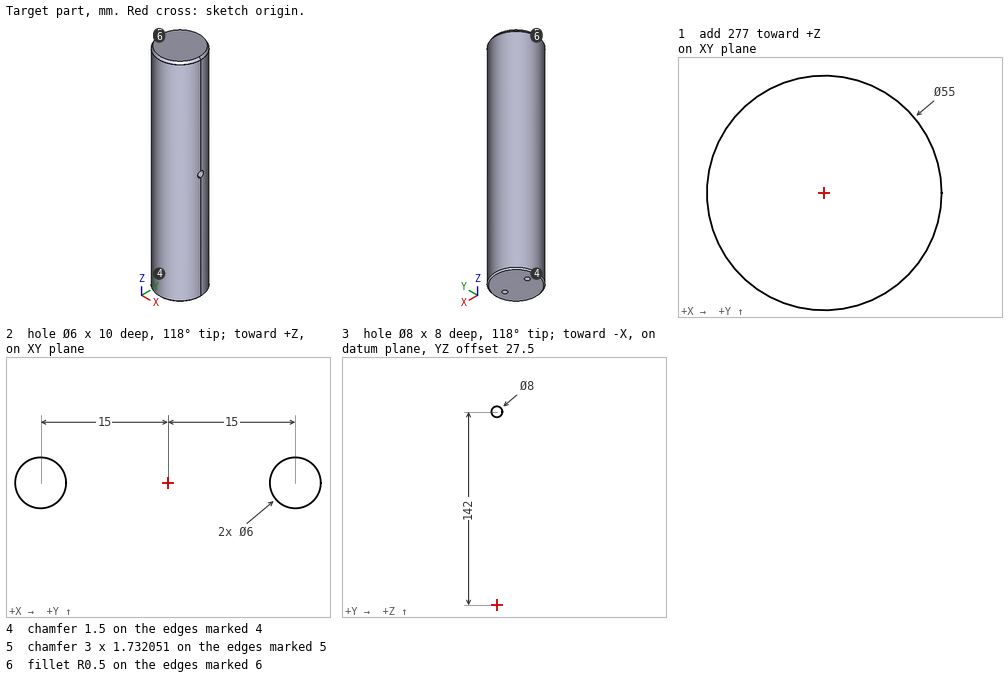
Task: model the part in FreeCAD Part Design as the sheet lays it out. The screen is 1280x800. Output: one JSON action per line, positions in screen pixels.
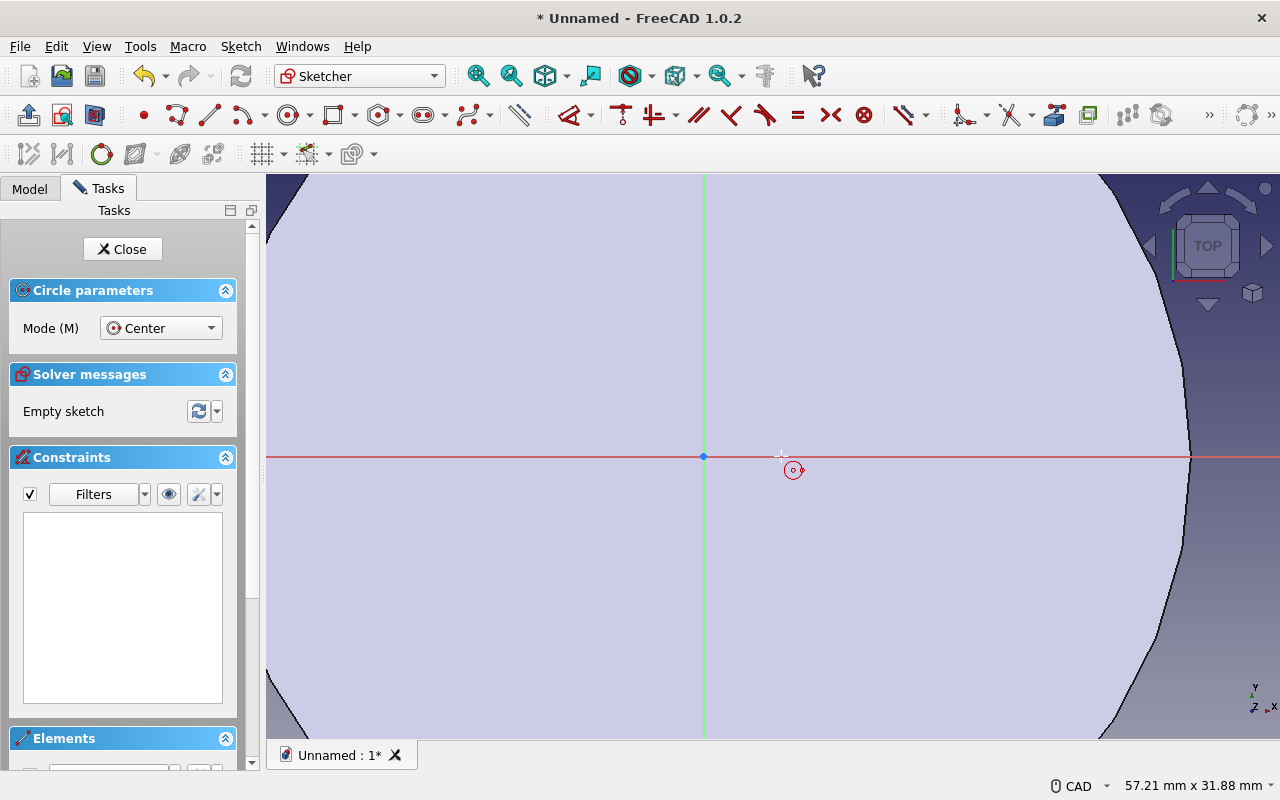
{"action": "left_click", "coordinate": [969, 456]}
{"action": "left_click", "coordinate": [1007, 419]}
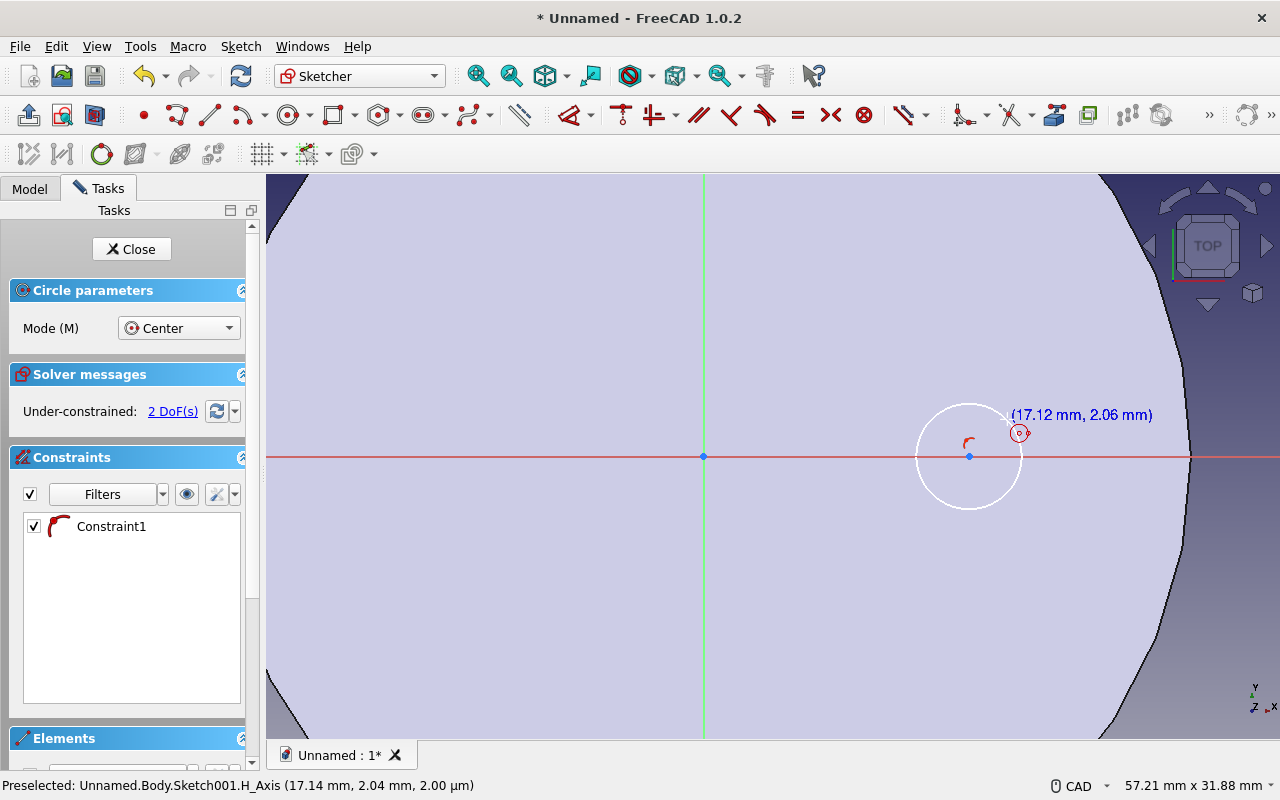
{"action": "left_click", "coordinate": [438, 456]}
{"action": "left_click", "coordinate": [475, 419]}
{"action": "key", "text": "Escape"}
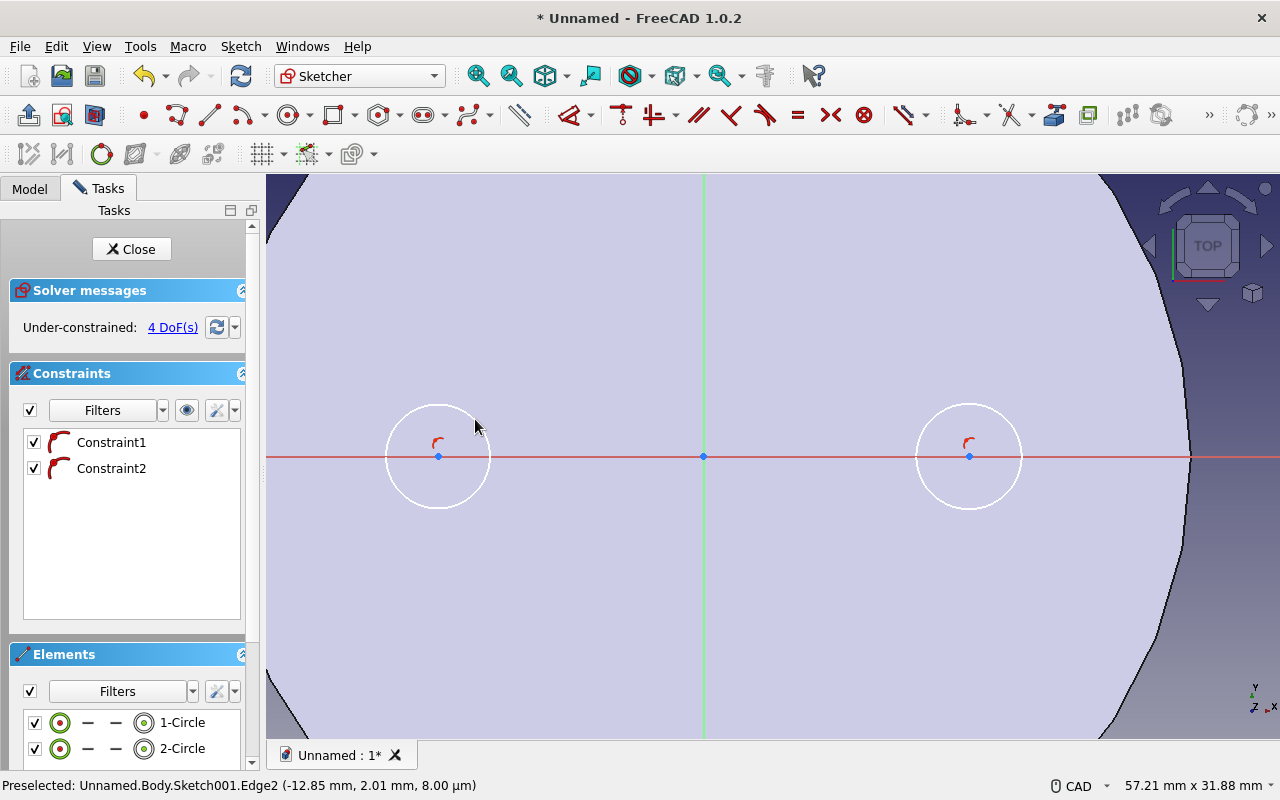
{"action": "left_click", "coordinate": [1006, 419]}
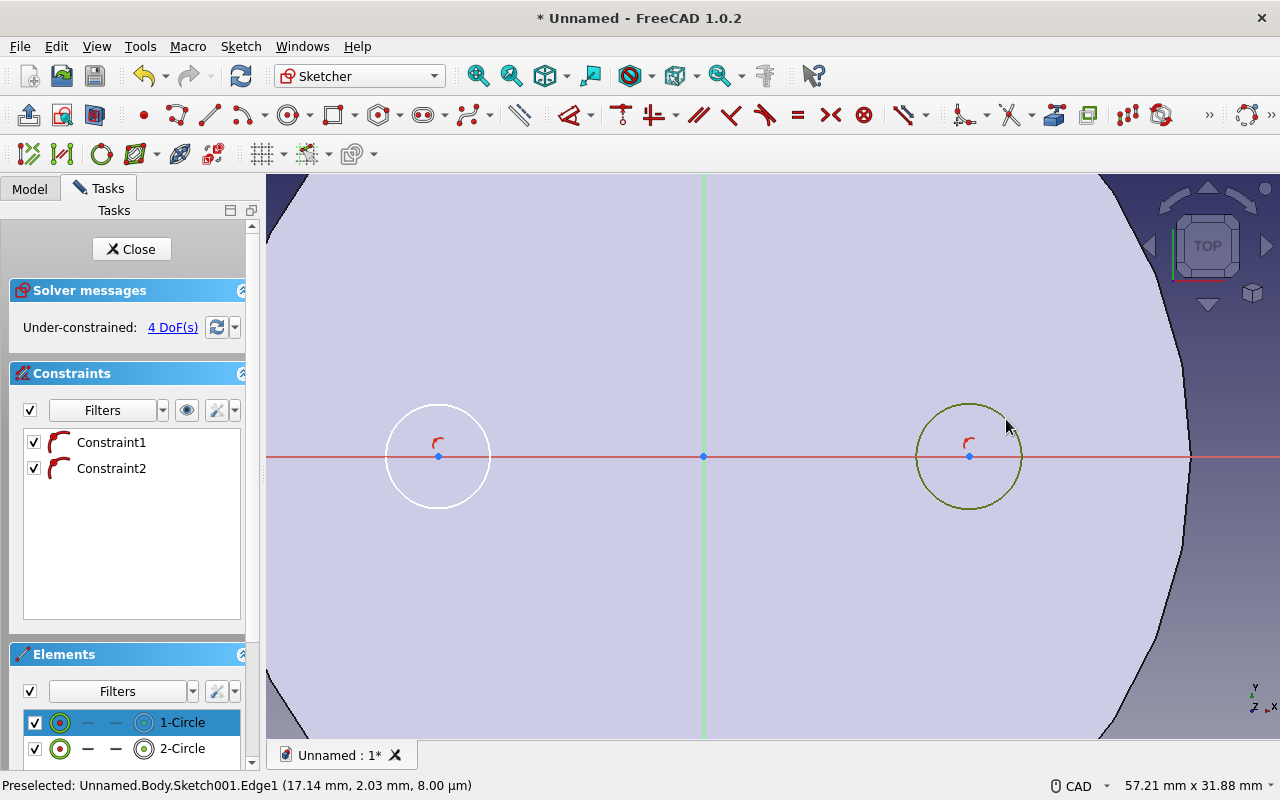
{"action": "left_click", "coordinate": [475, 420]}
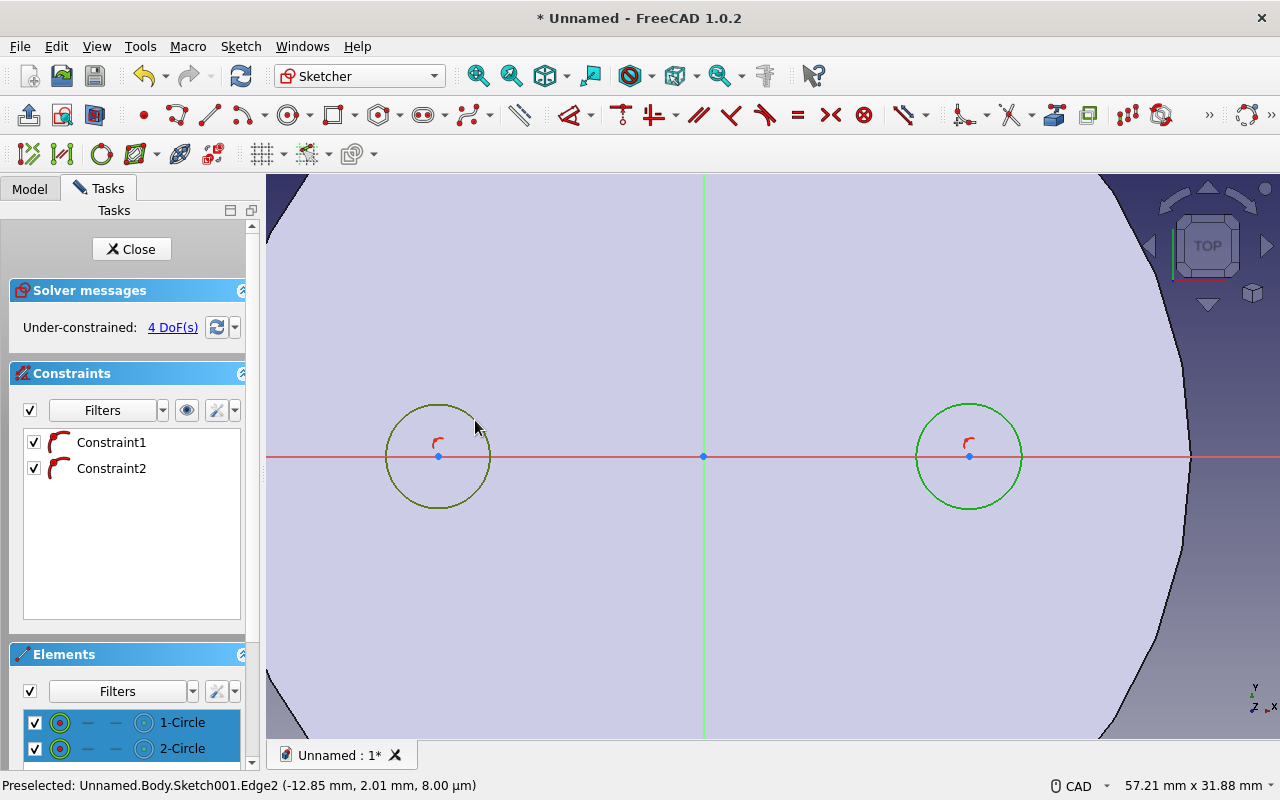
{"action": "left_click", "coordinate": [798, 116]}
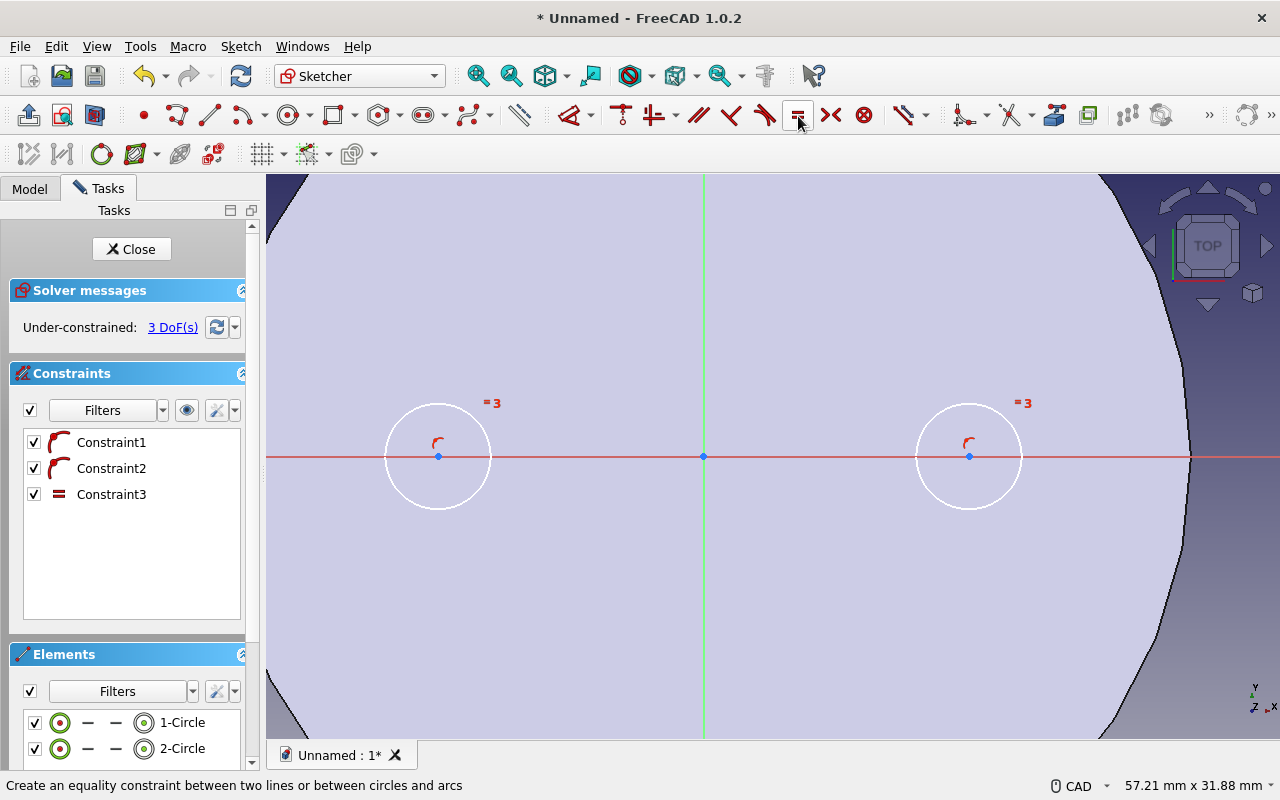
{"action": "key", "text": "d"}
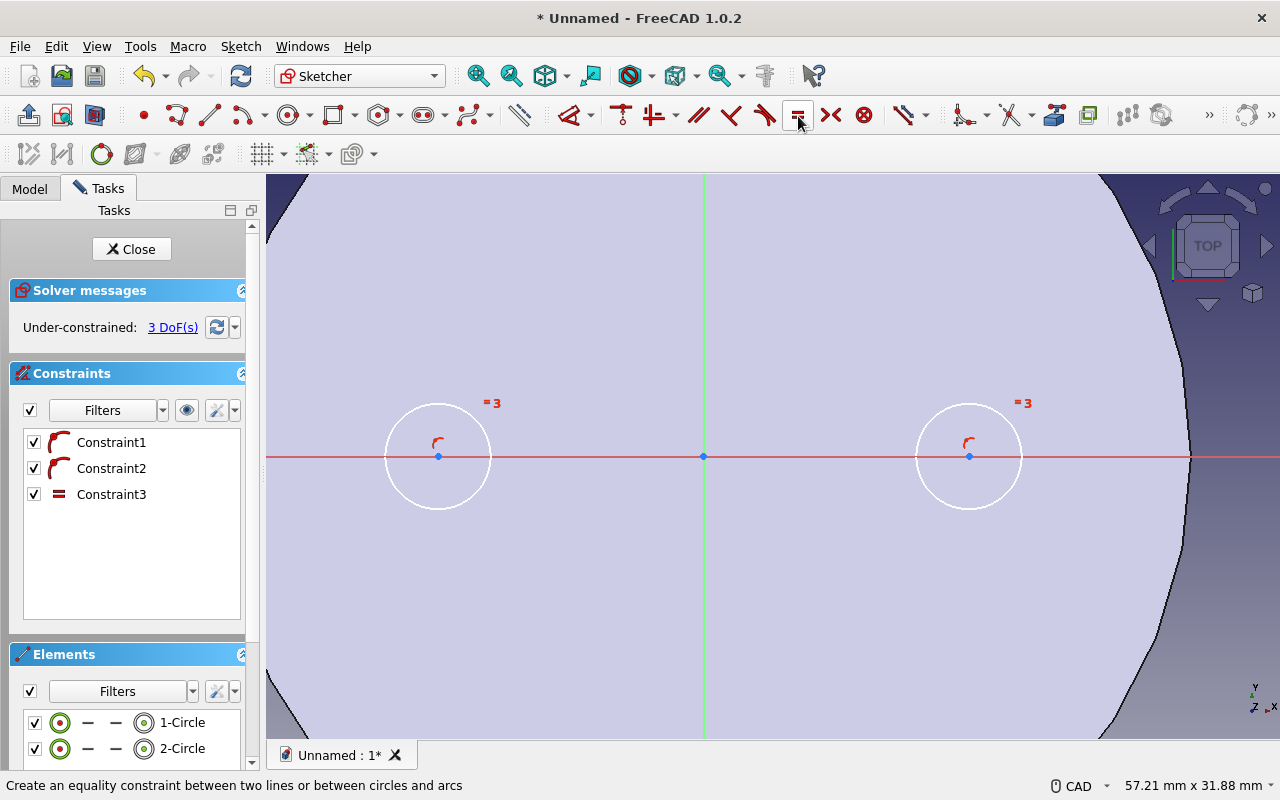
{"action": "left_click", "coordinate": [1006, 419]}
{"action": "left_click", "coordinate": [1028, 396]}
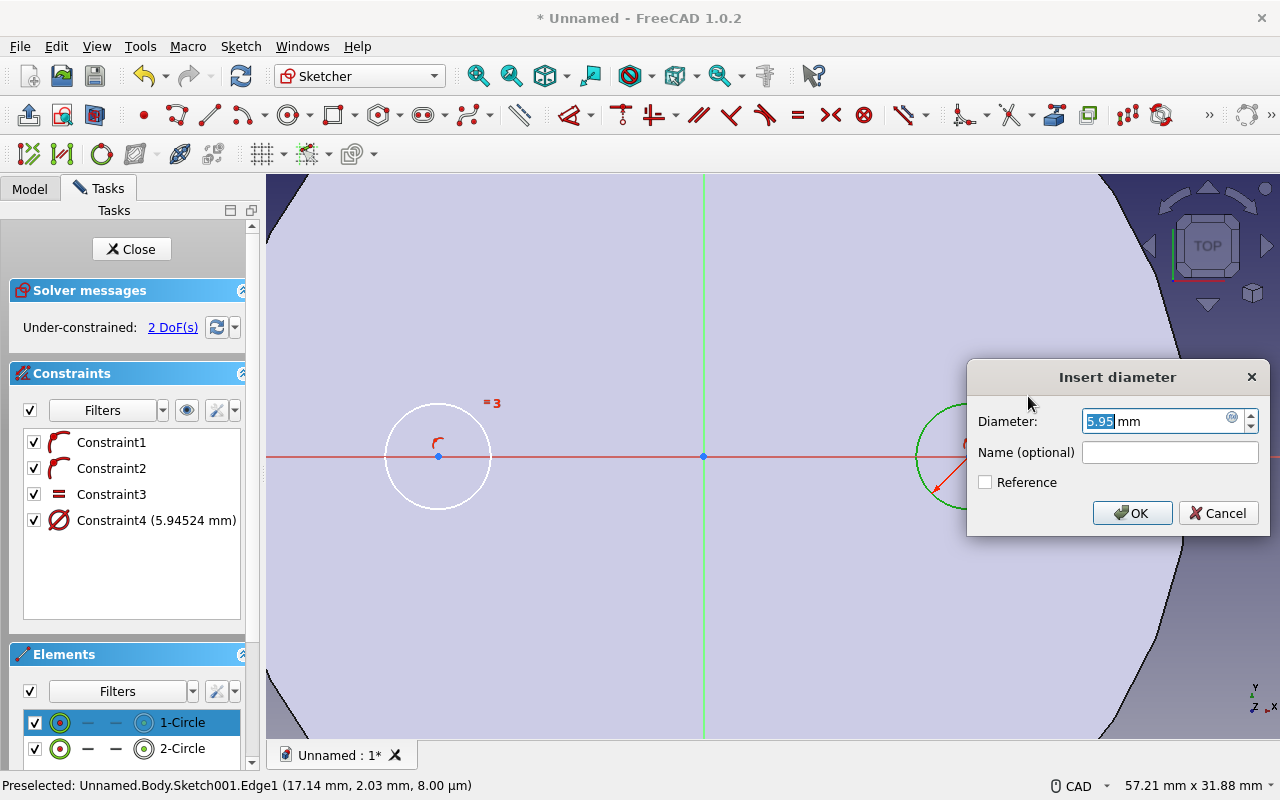
{"action": "type", "text": "6"}
{"action": "key", "text": "Return"}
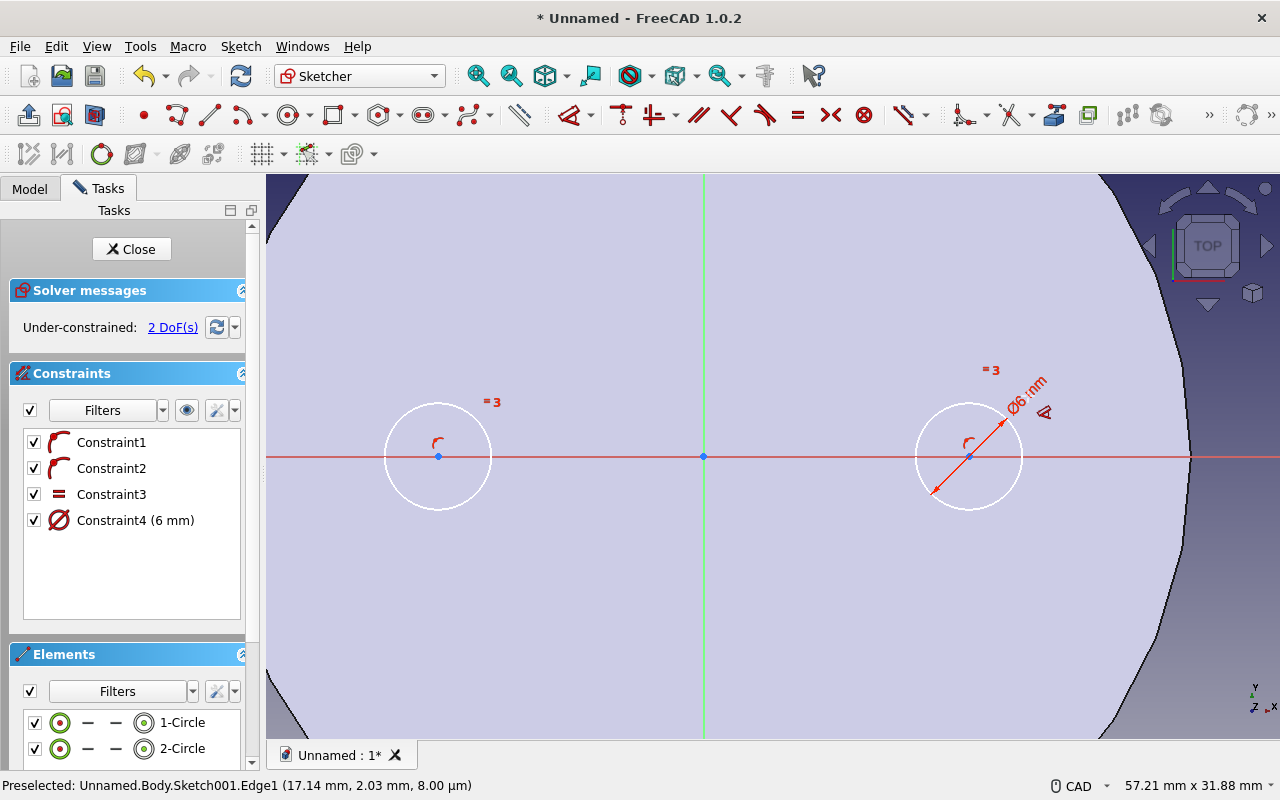
{"action": "left_click", "coordinate": [969, 456]}
{"action": "left_click", "coordinate": [836, 490]}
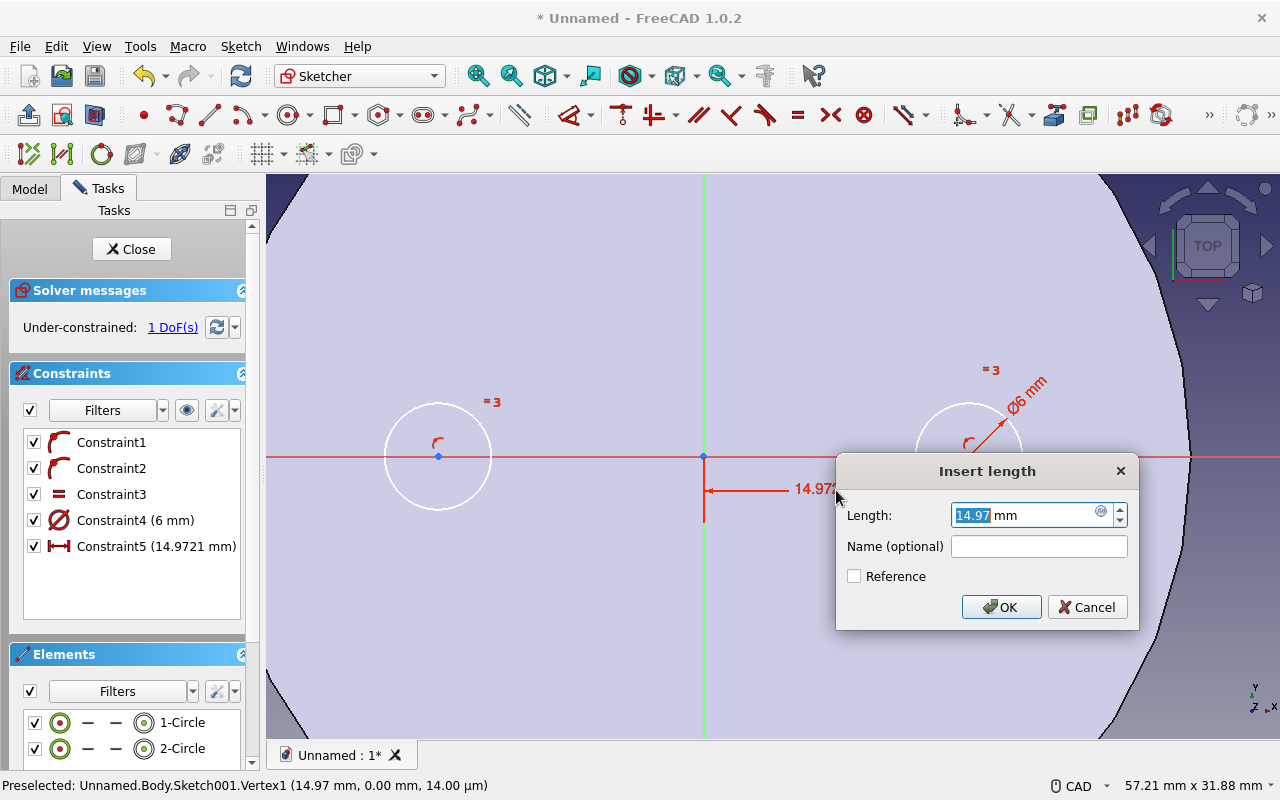
{"action": "type", "text": "15"}
{"action": "key", "text": "Return"}